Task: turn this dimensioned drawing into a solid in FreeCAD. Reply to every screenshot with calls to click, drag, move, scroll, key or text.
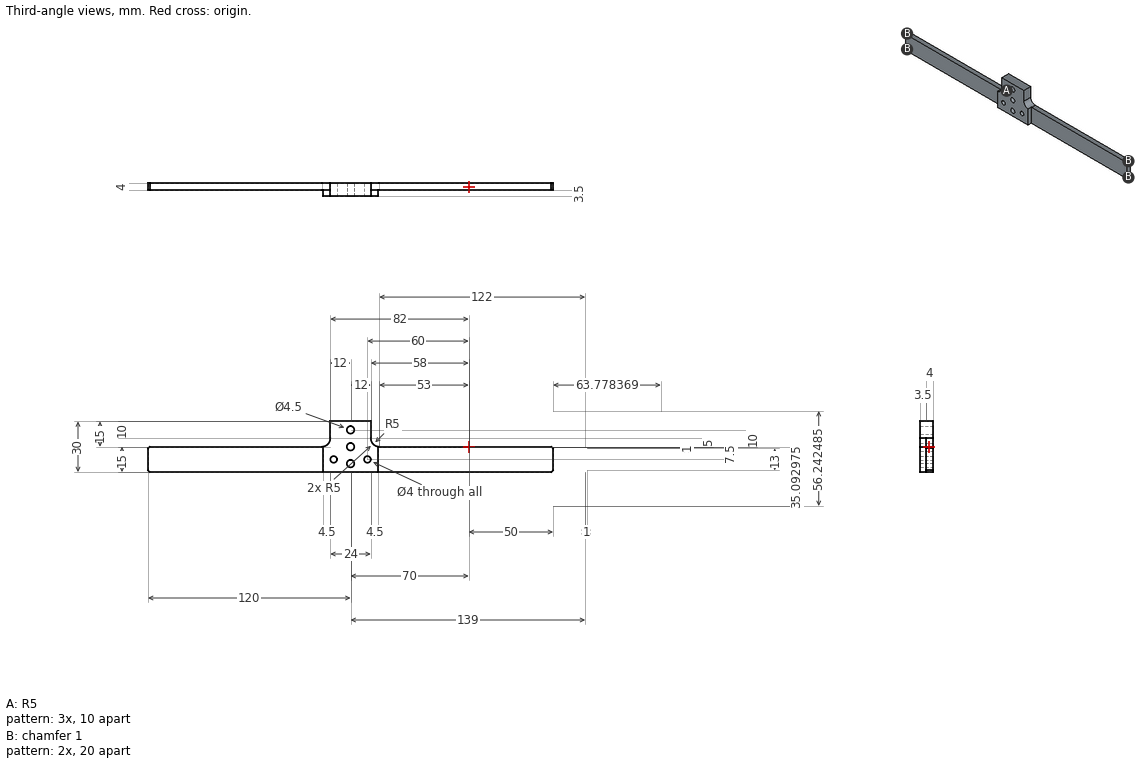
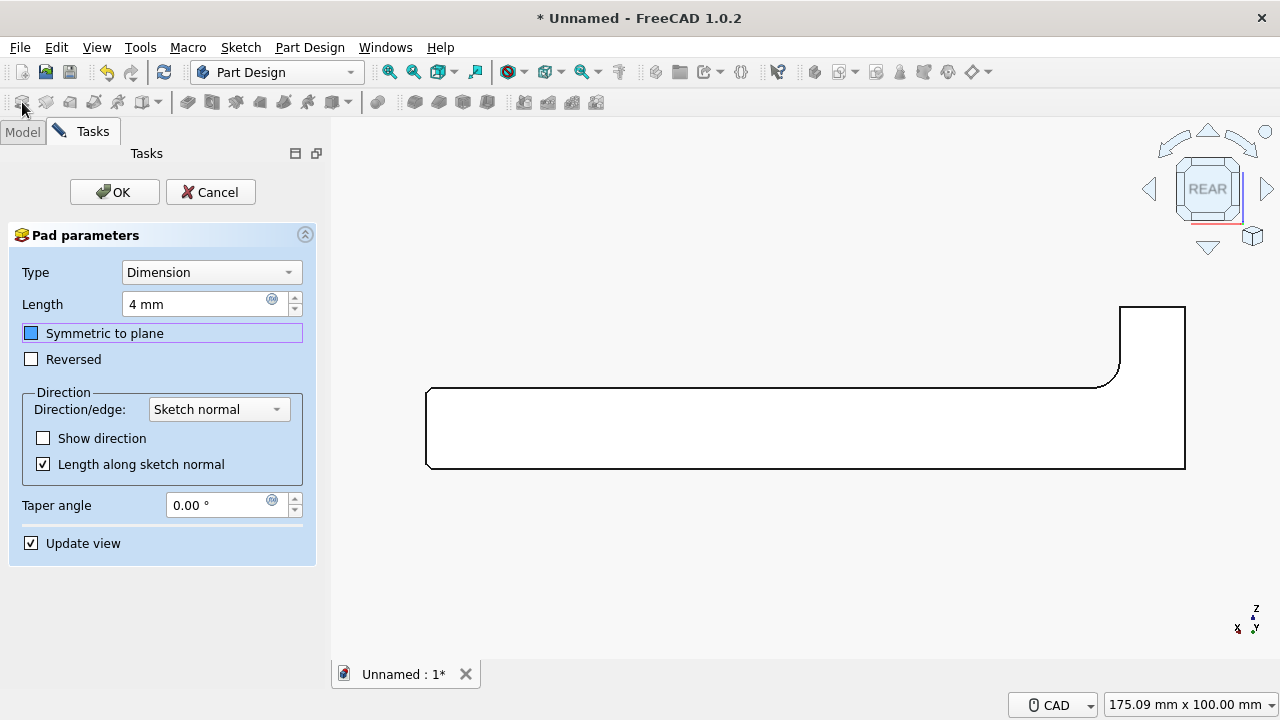
click(30, 359)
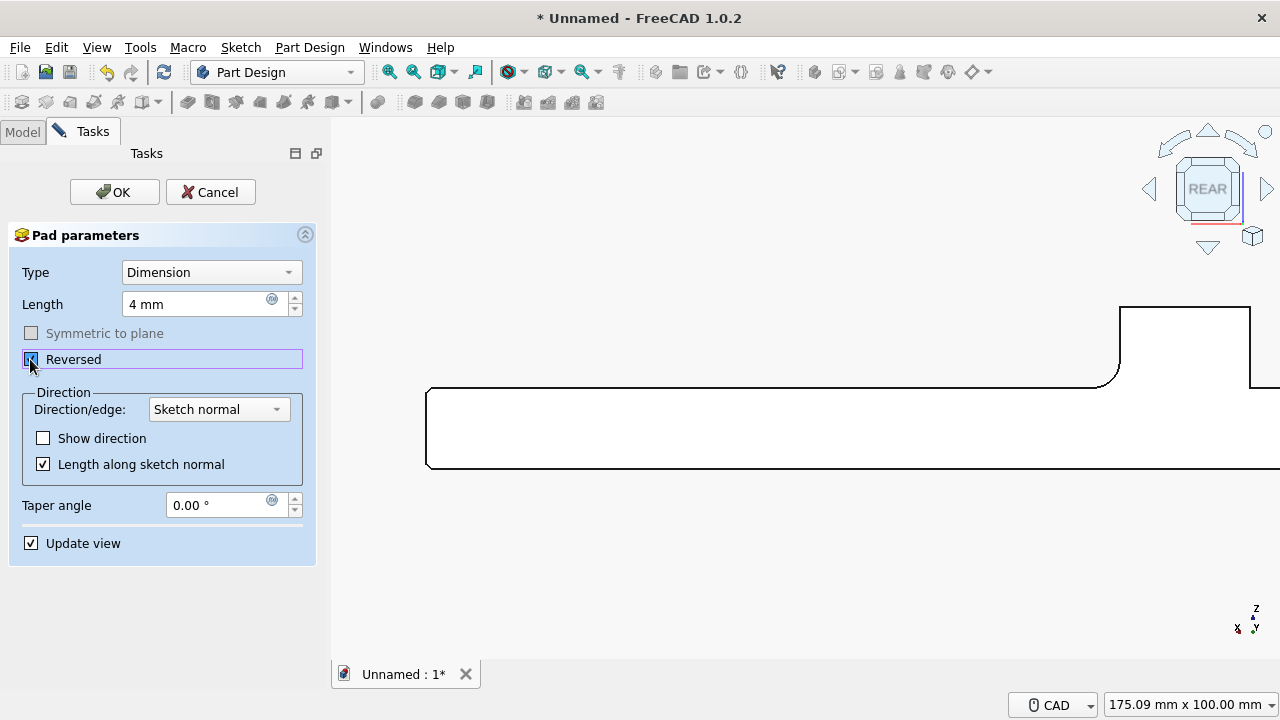
click(115, 192)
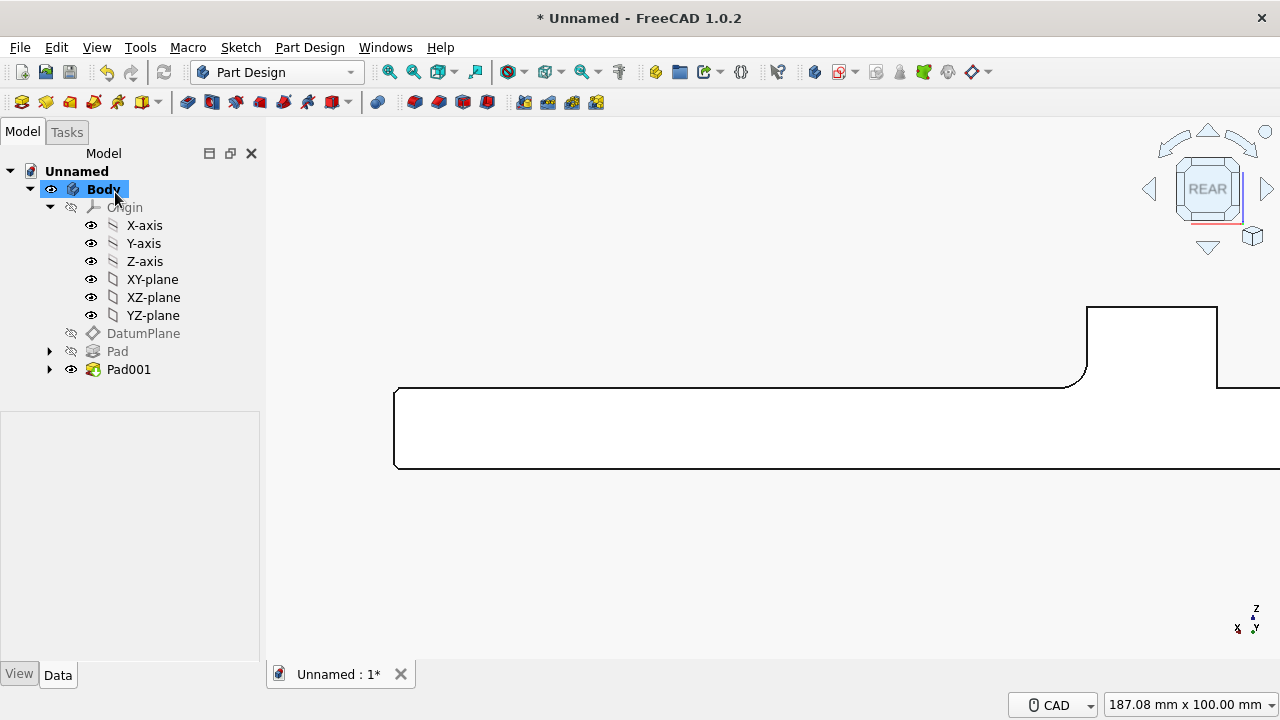
click(390, 72)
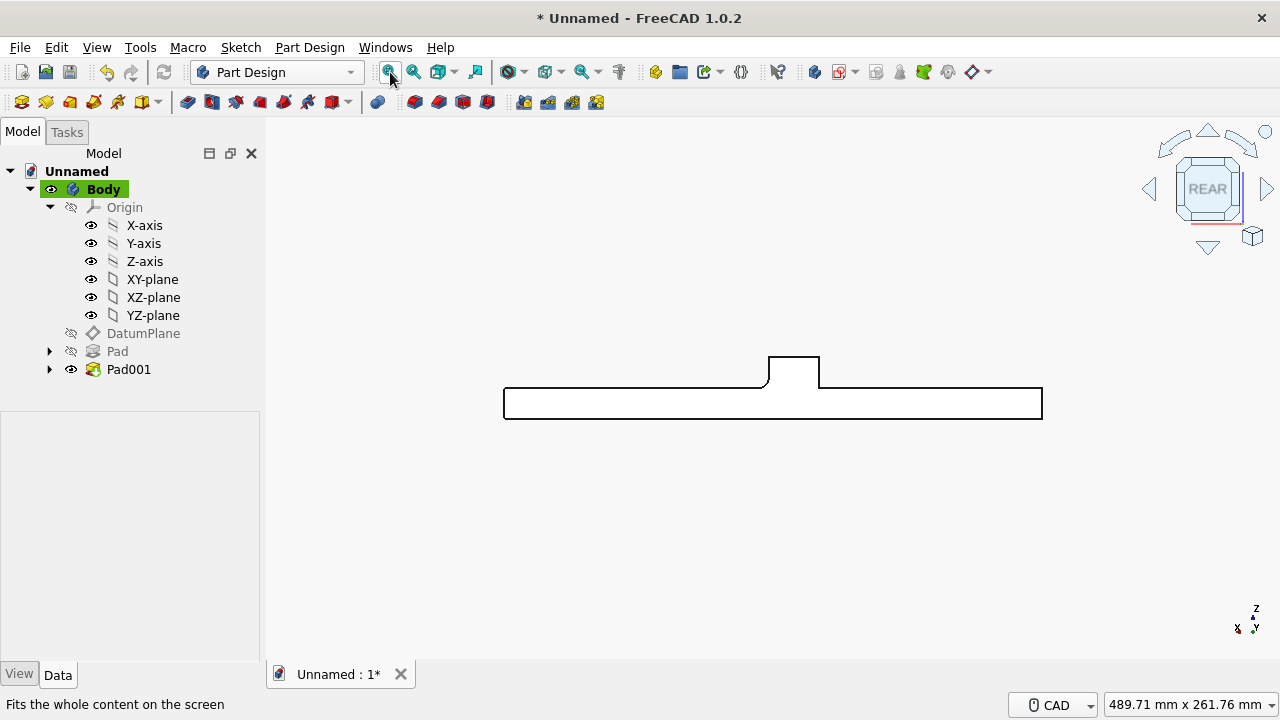
scroll(819, 387, up, 8)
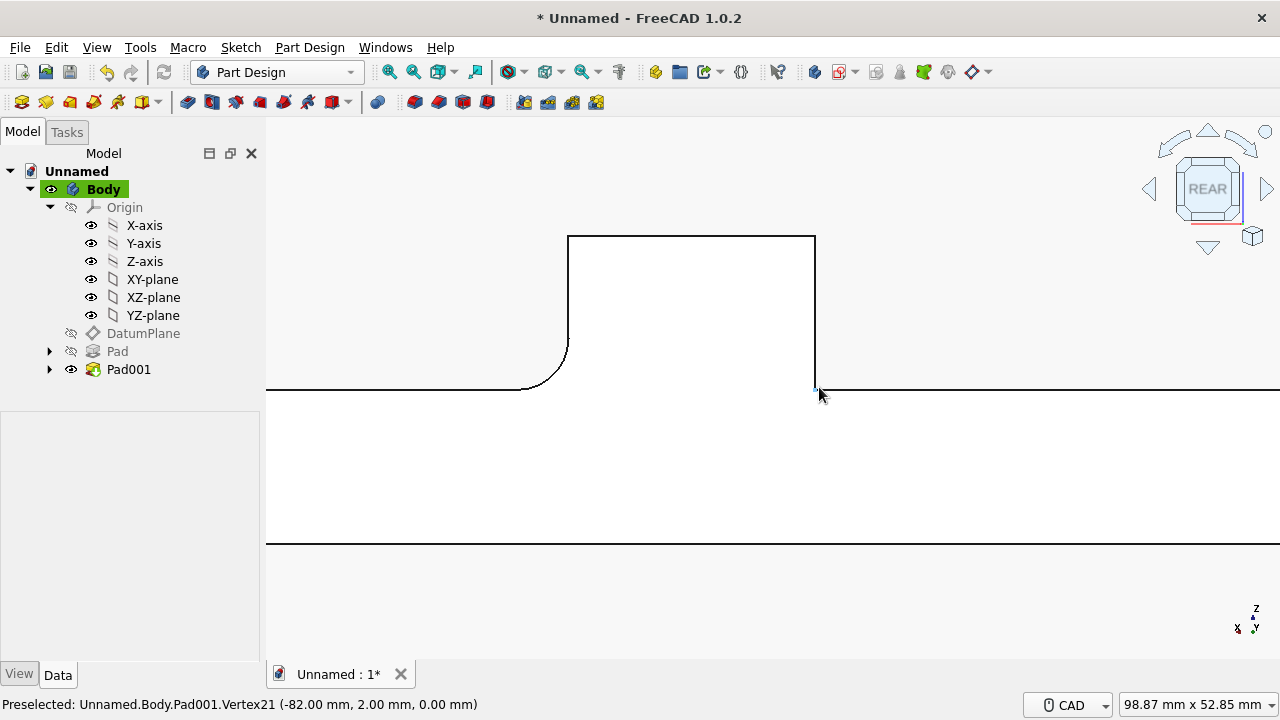
click(390, 72)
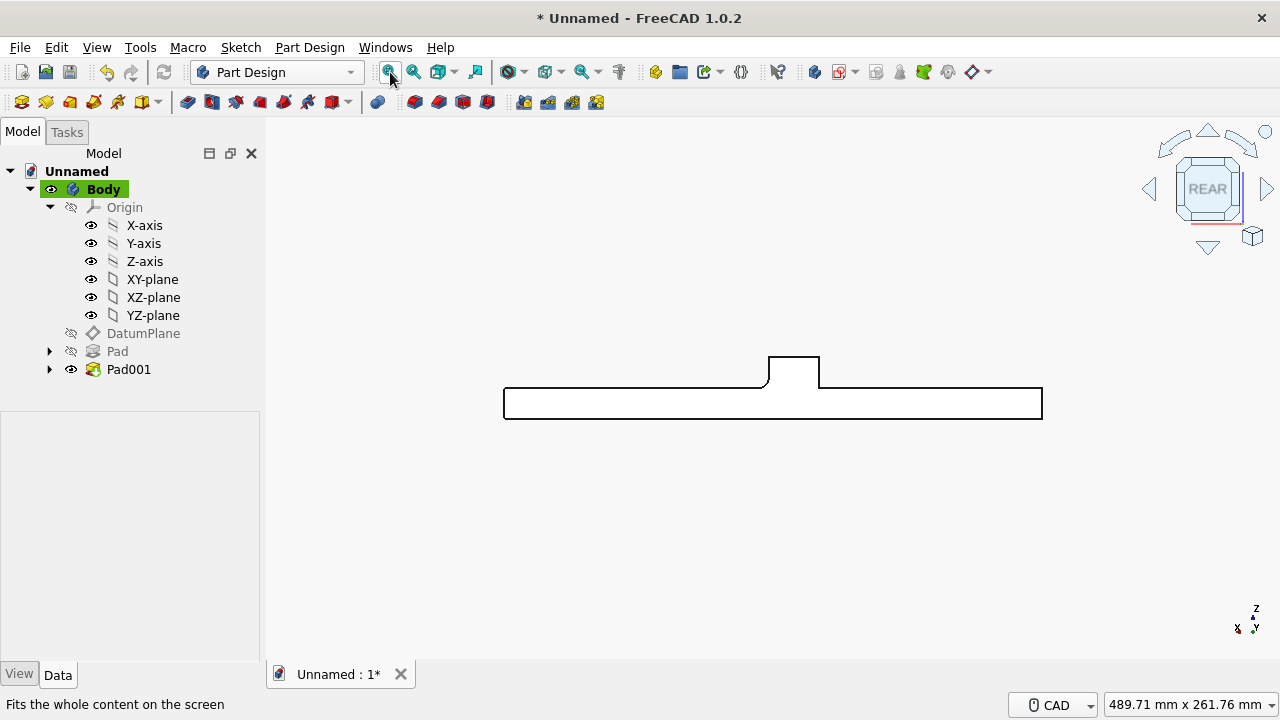
key(0)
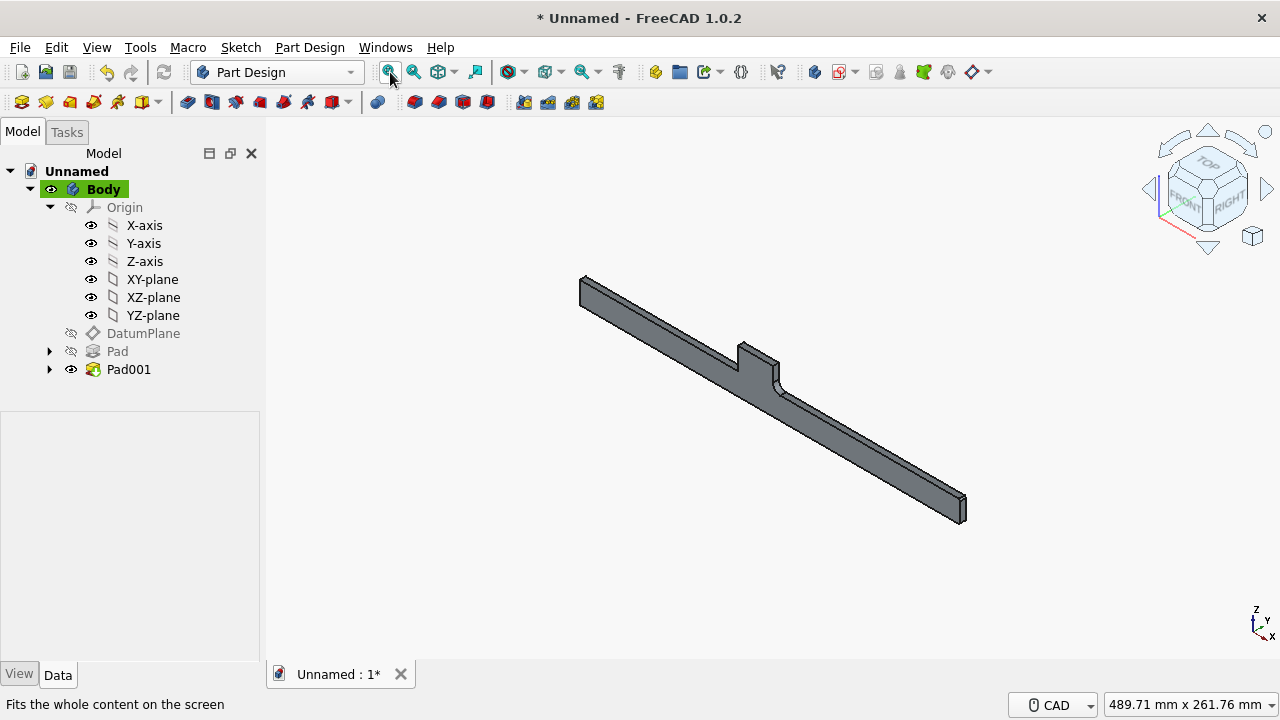
scroll(741, 368, up, 8)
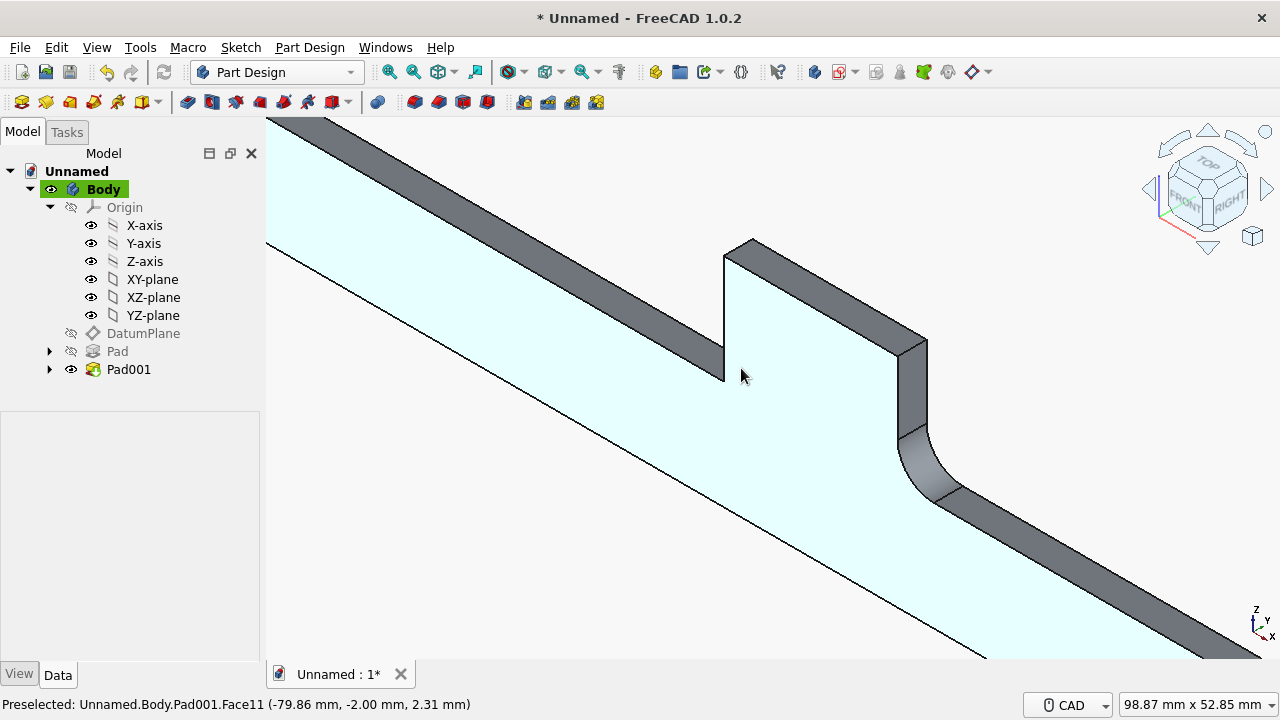
click(390, 72)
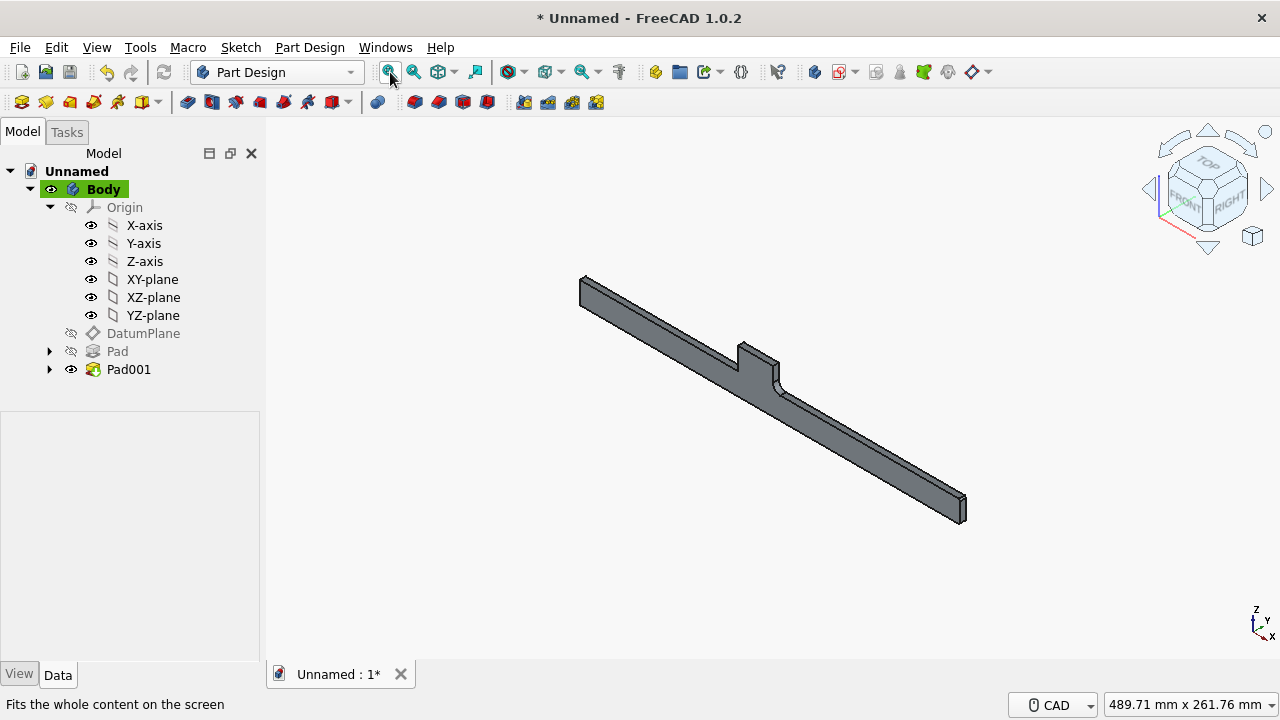
key(2)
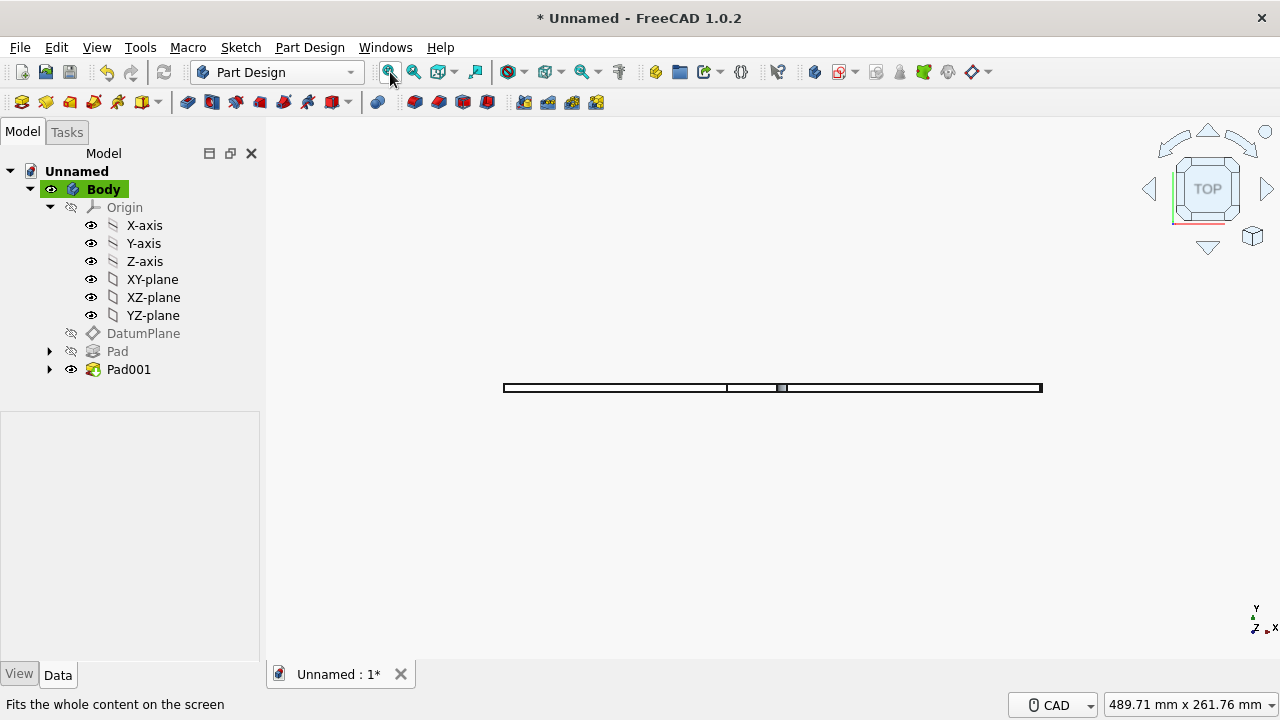
scroll(727, 387, up, 8)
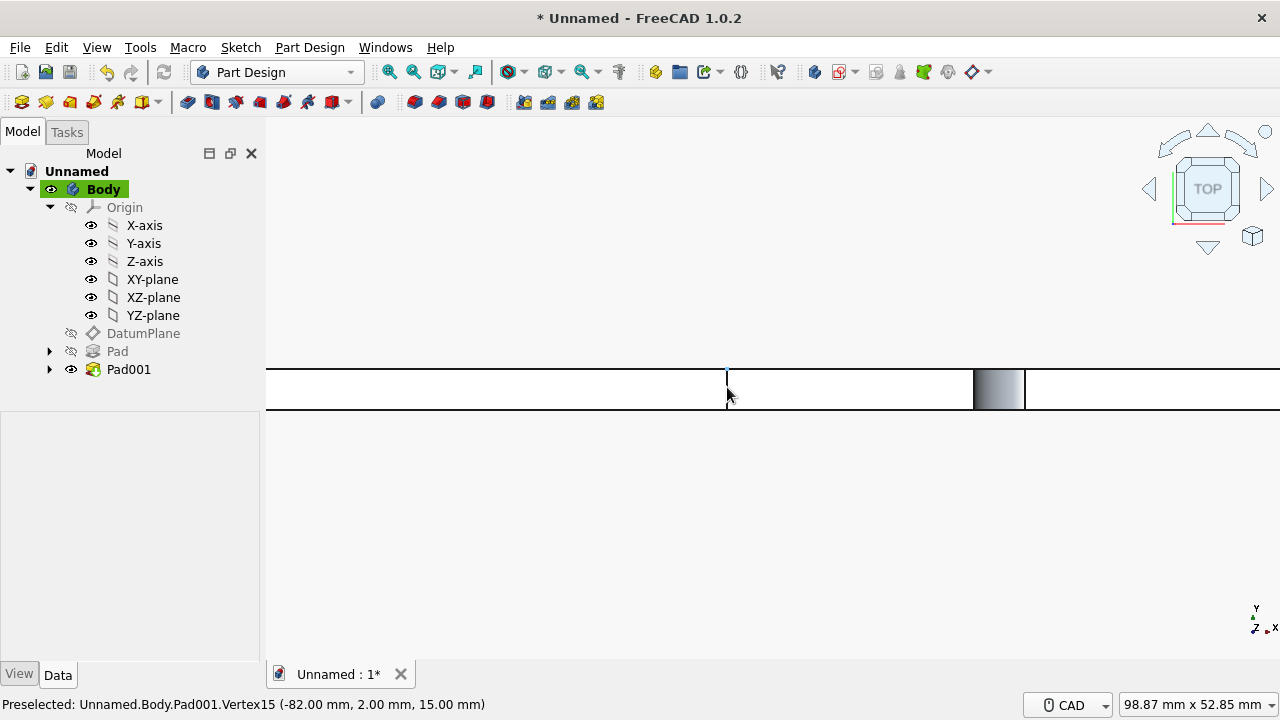
click(390, 72)